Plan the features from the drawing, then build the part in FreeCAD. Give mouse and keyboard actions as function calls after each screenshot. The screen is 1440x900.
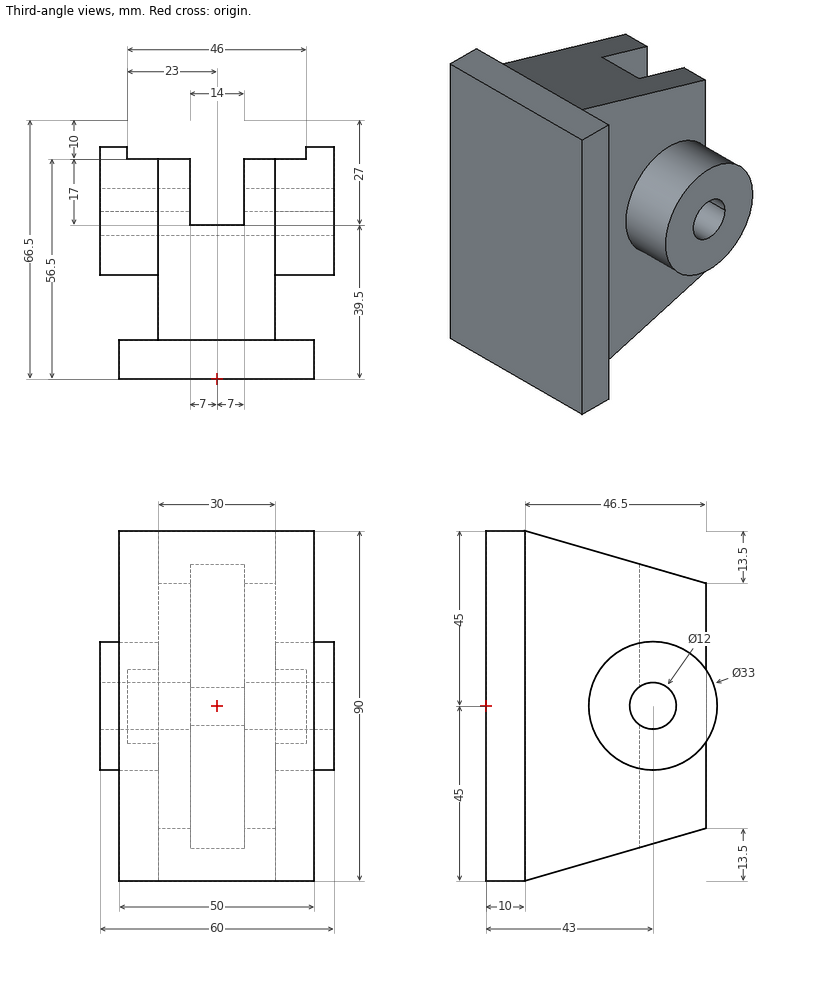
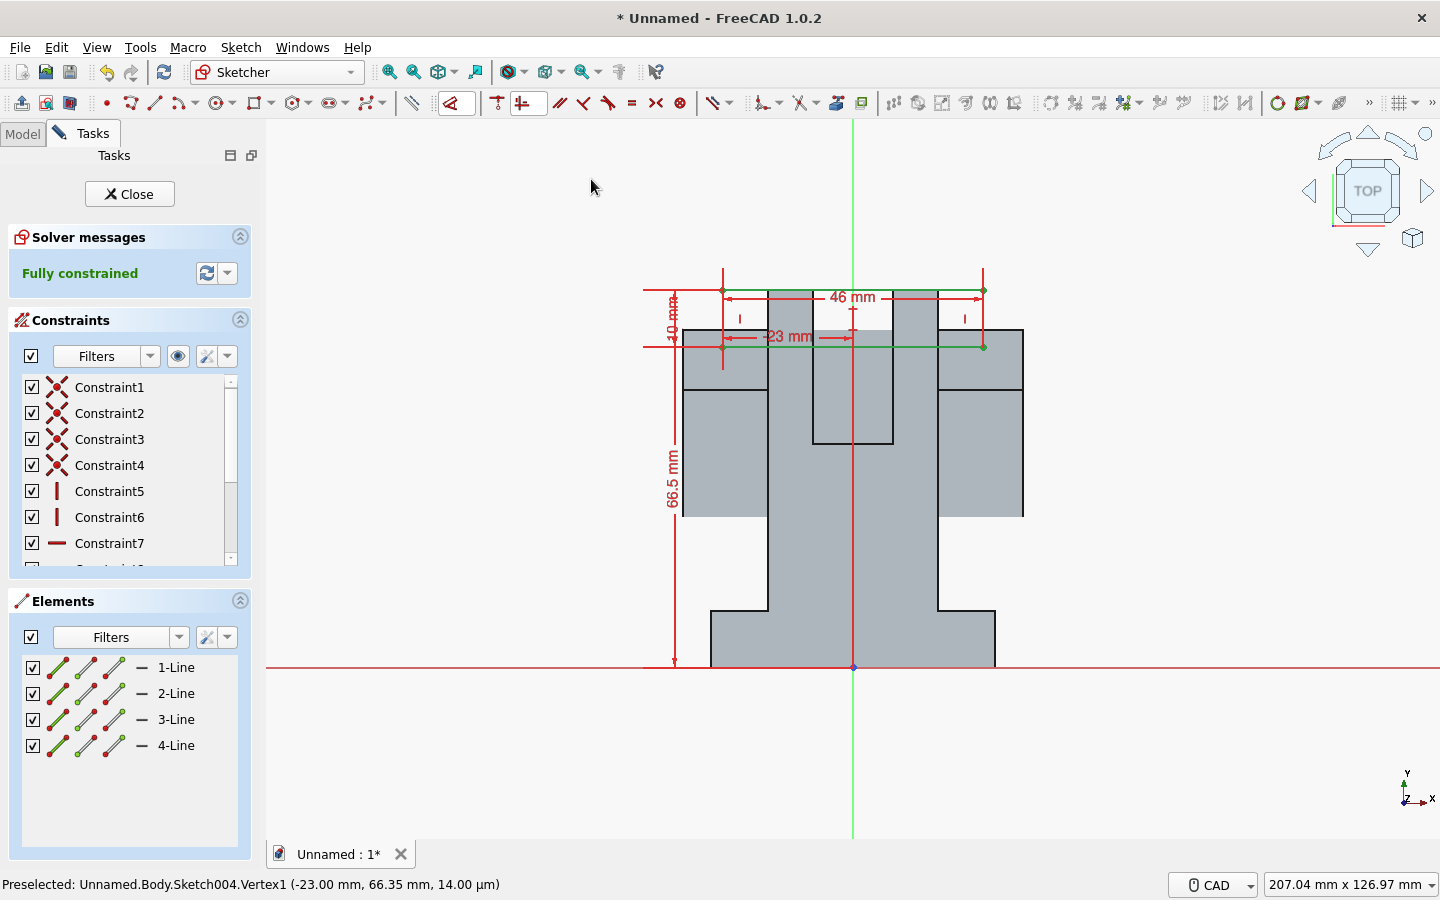
click(130, 194)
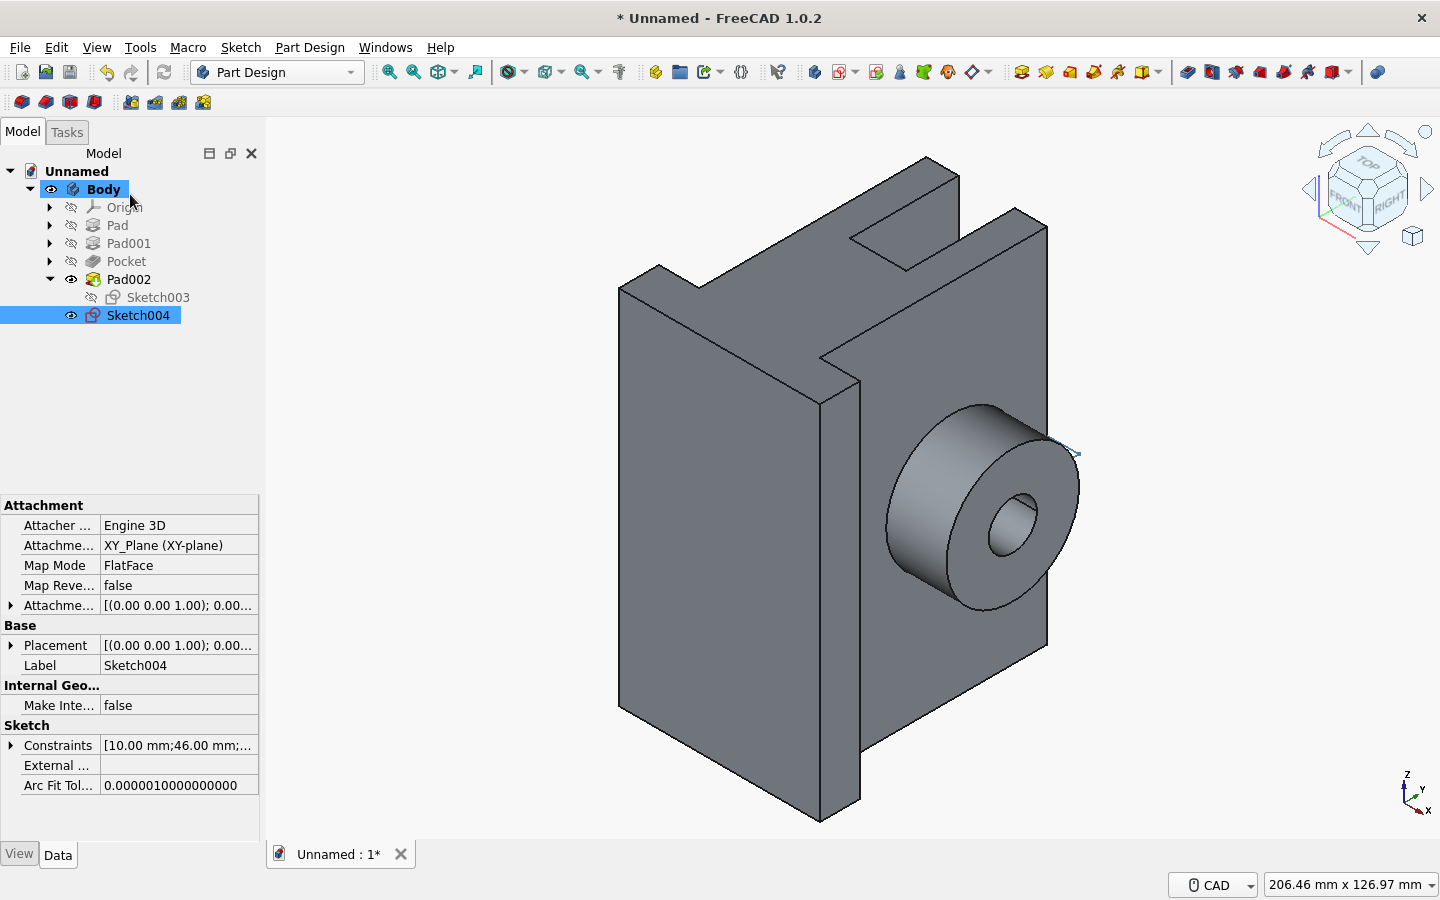
click(1188, 72)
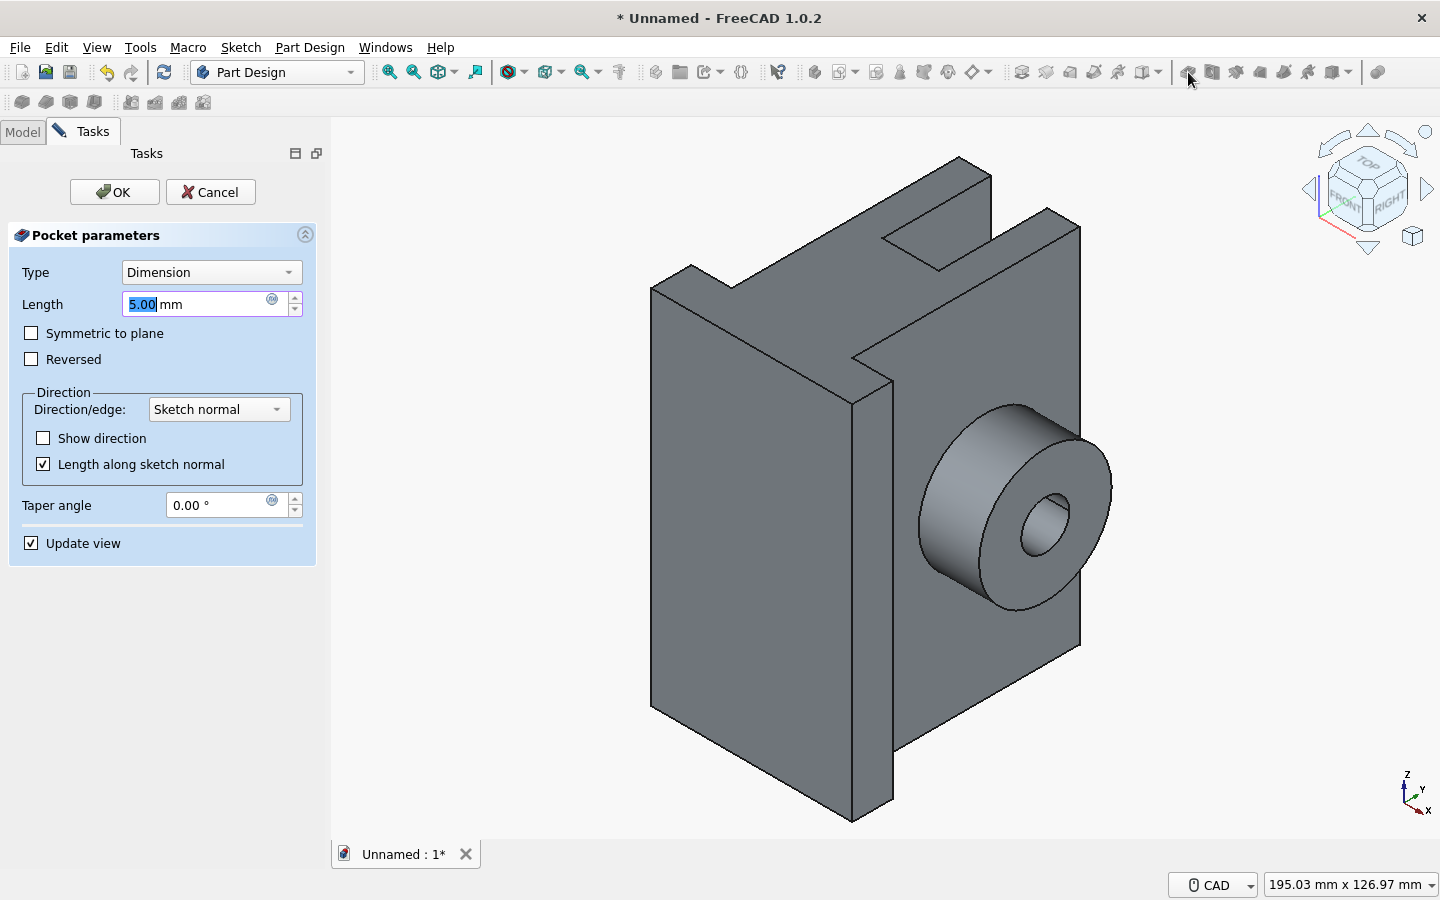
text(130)
key(Tab)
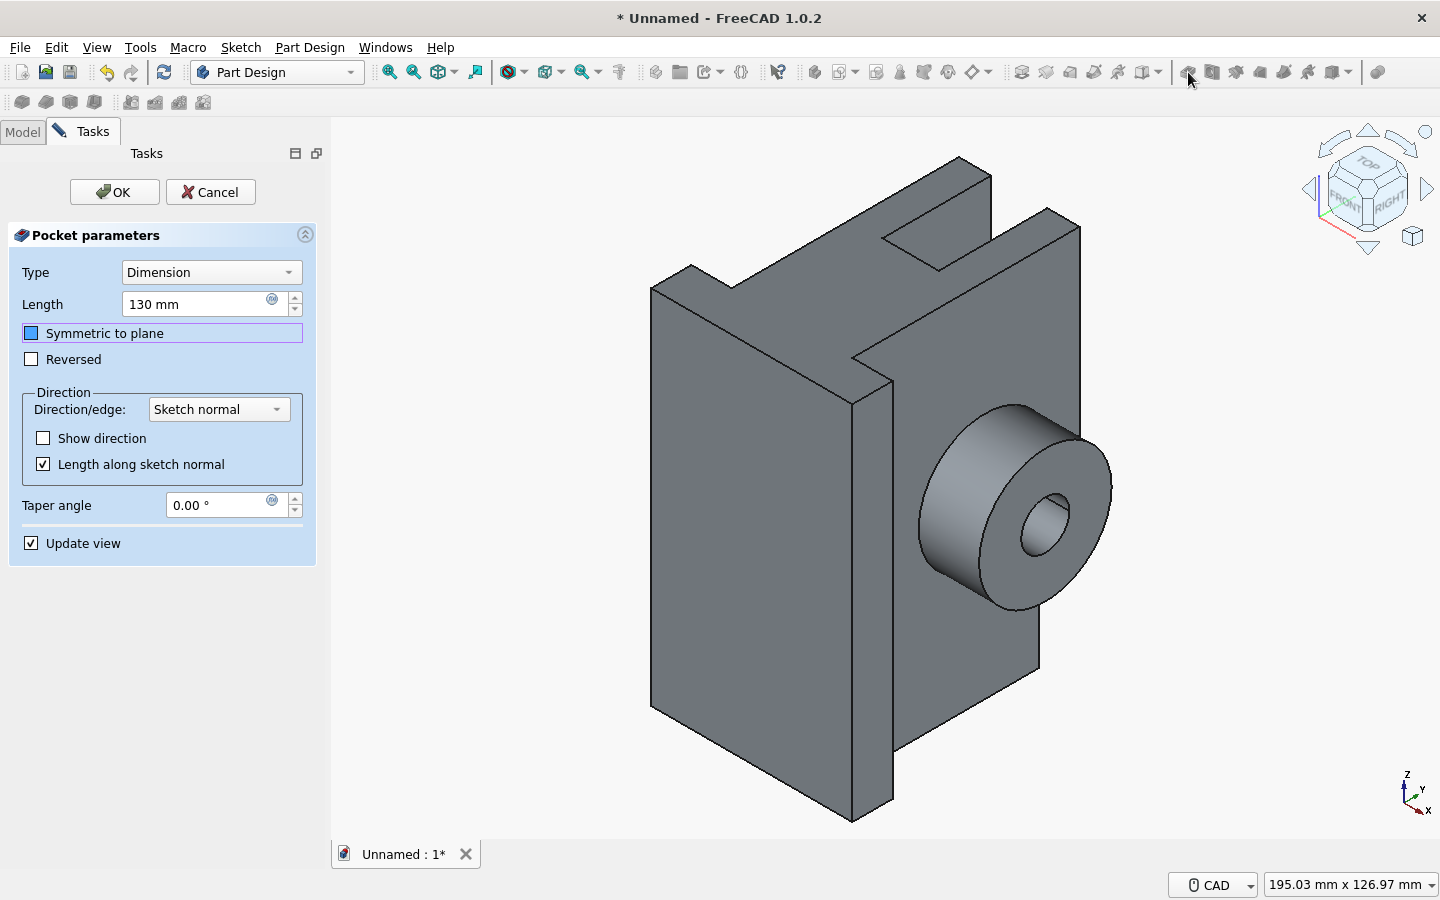
click(30, 333)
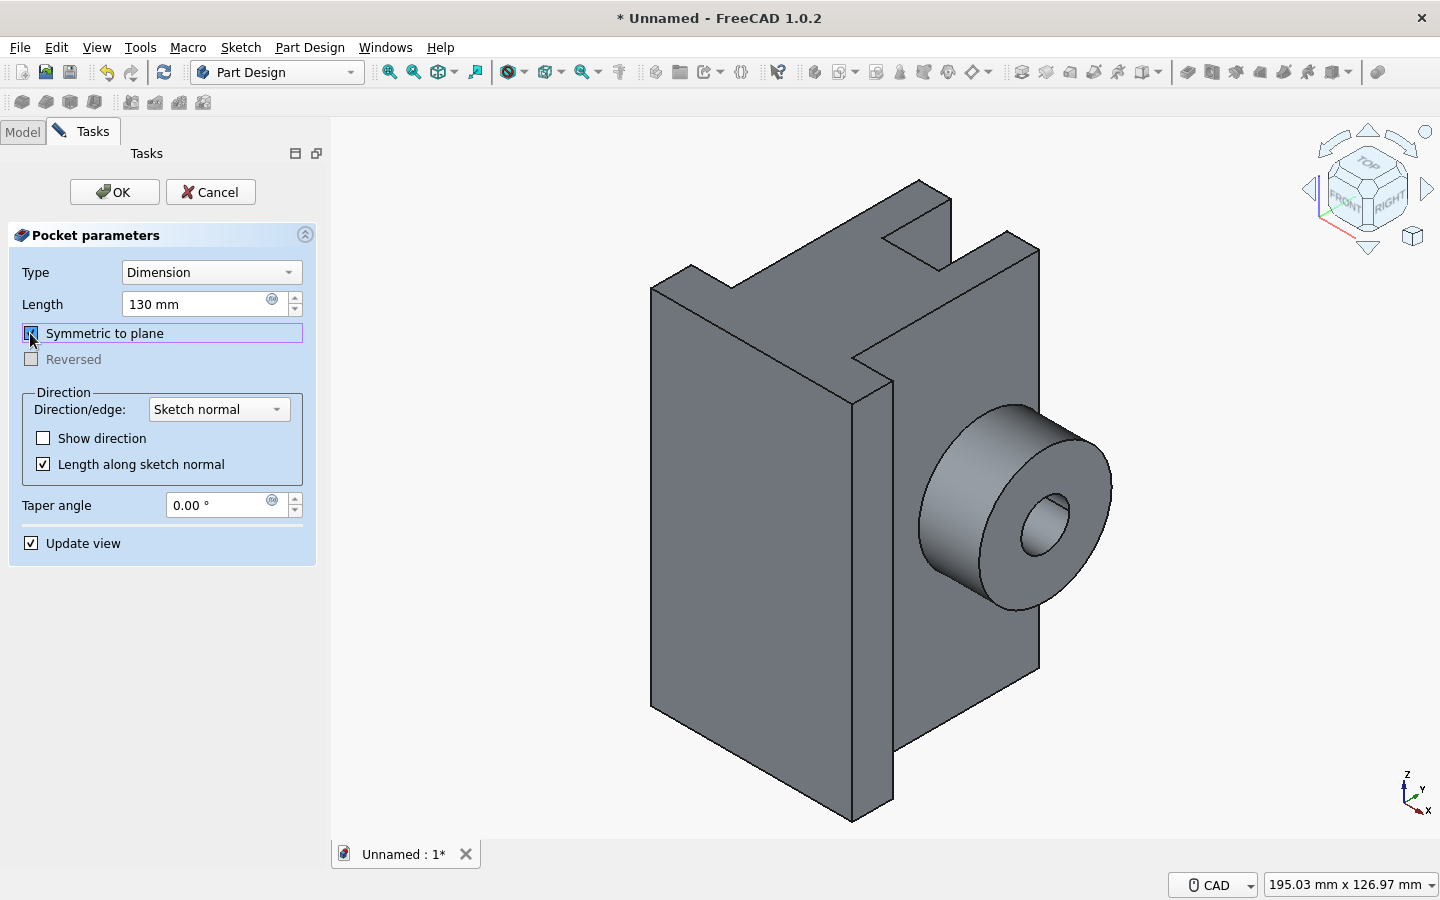
click(115, 192)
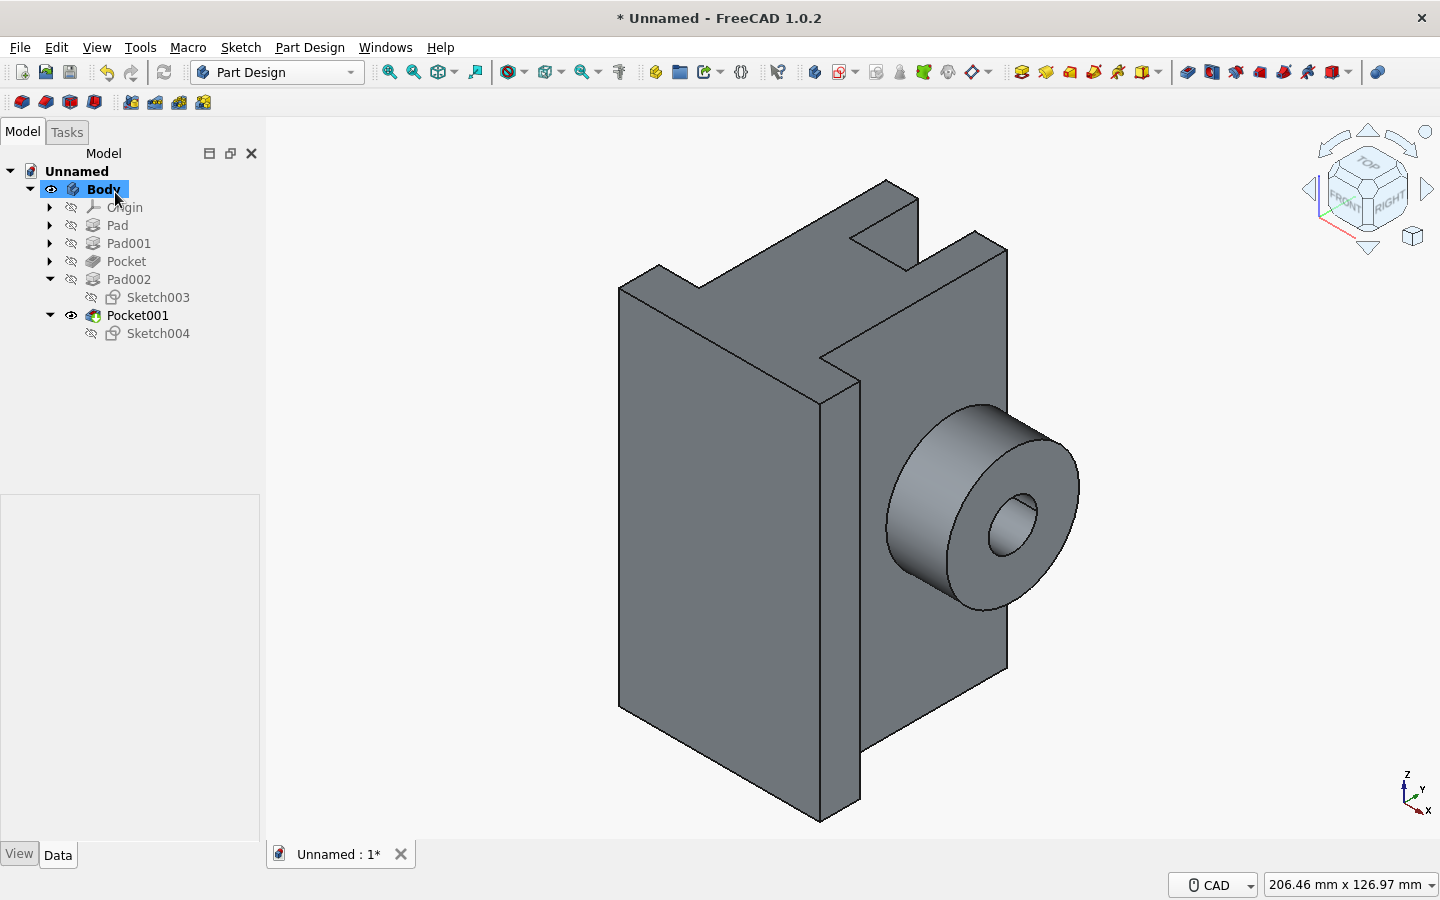
click(840, 72)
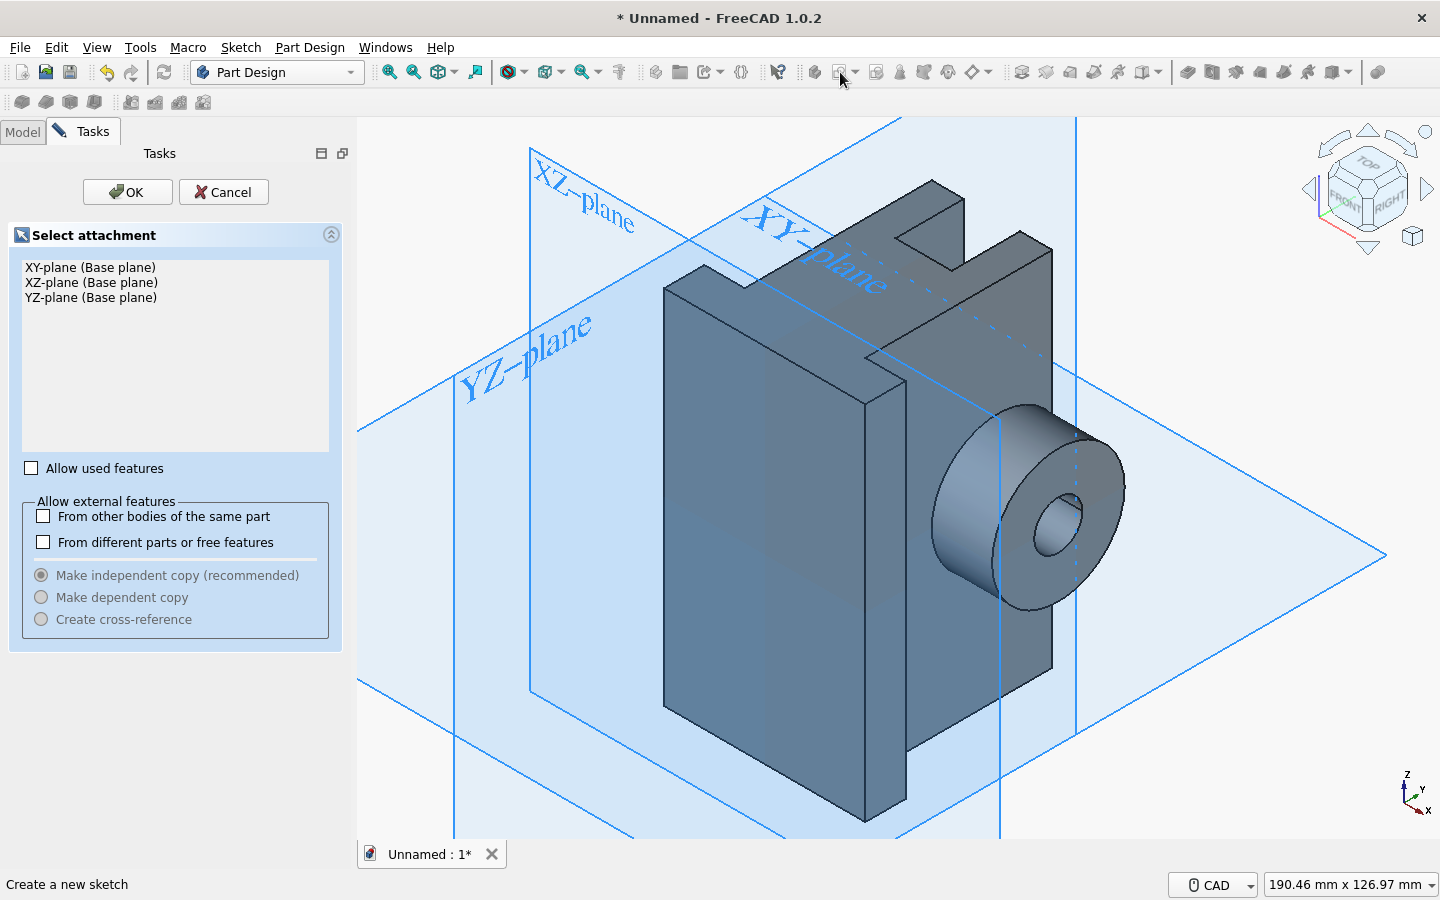
click(82, 298)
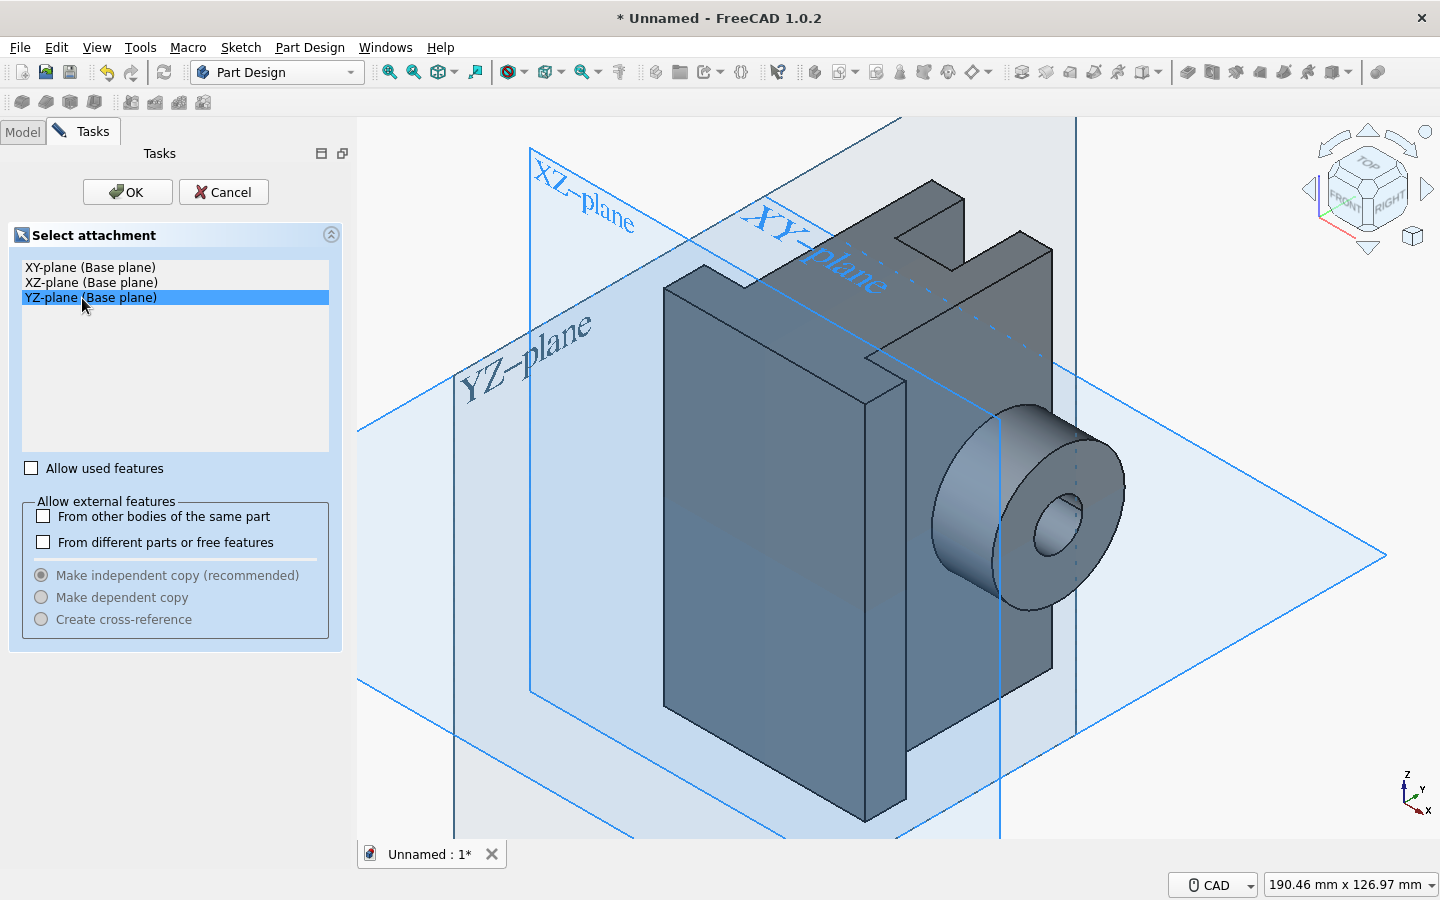
click(128, 192)